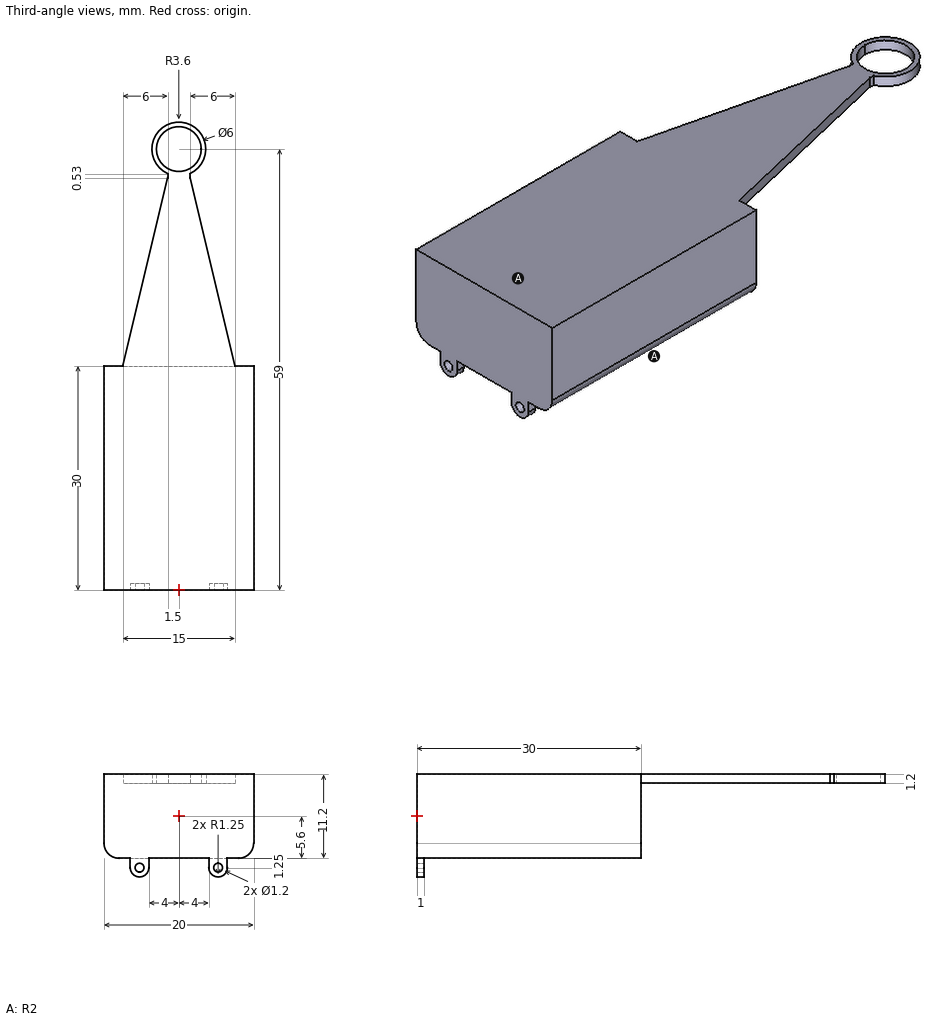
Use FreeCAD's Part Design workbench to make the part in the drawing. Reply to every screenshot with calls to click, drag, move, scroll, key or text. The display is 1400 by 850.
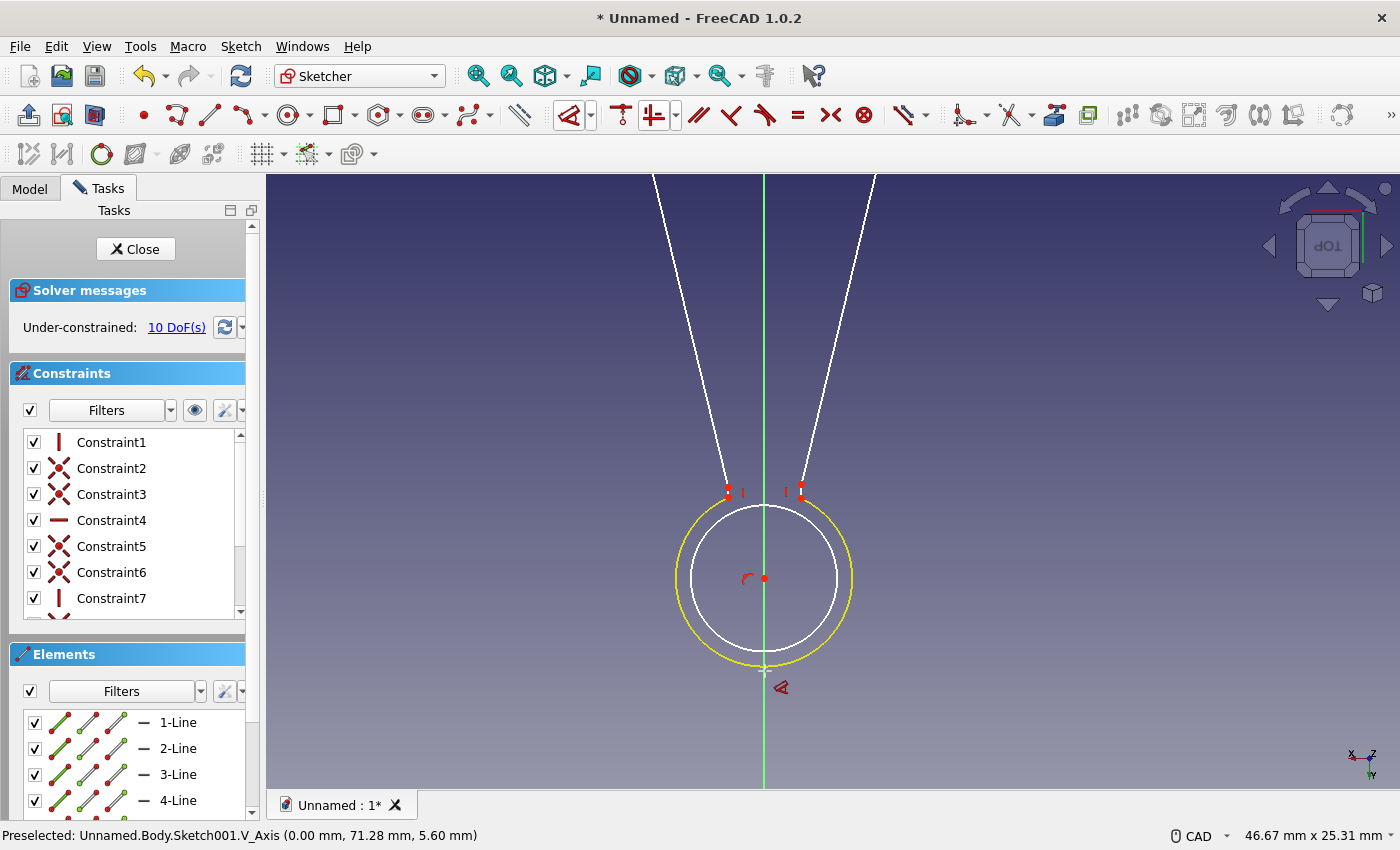
click(763, 667)
click(705, 684)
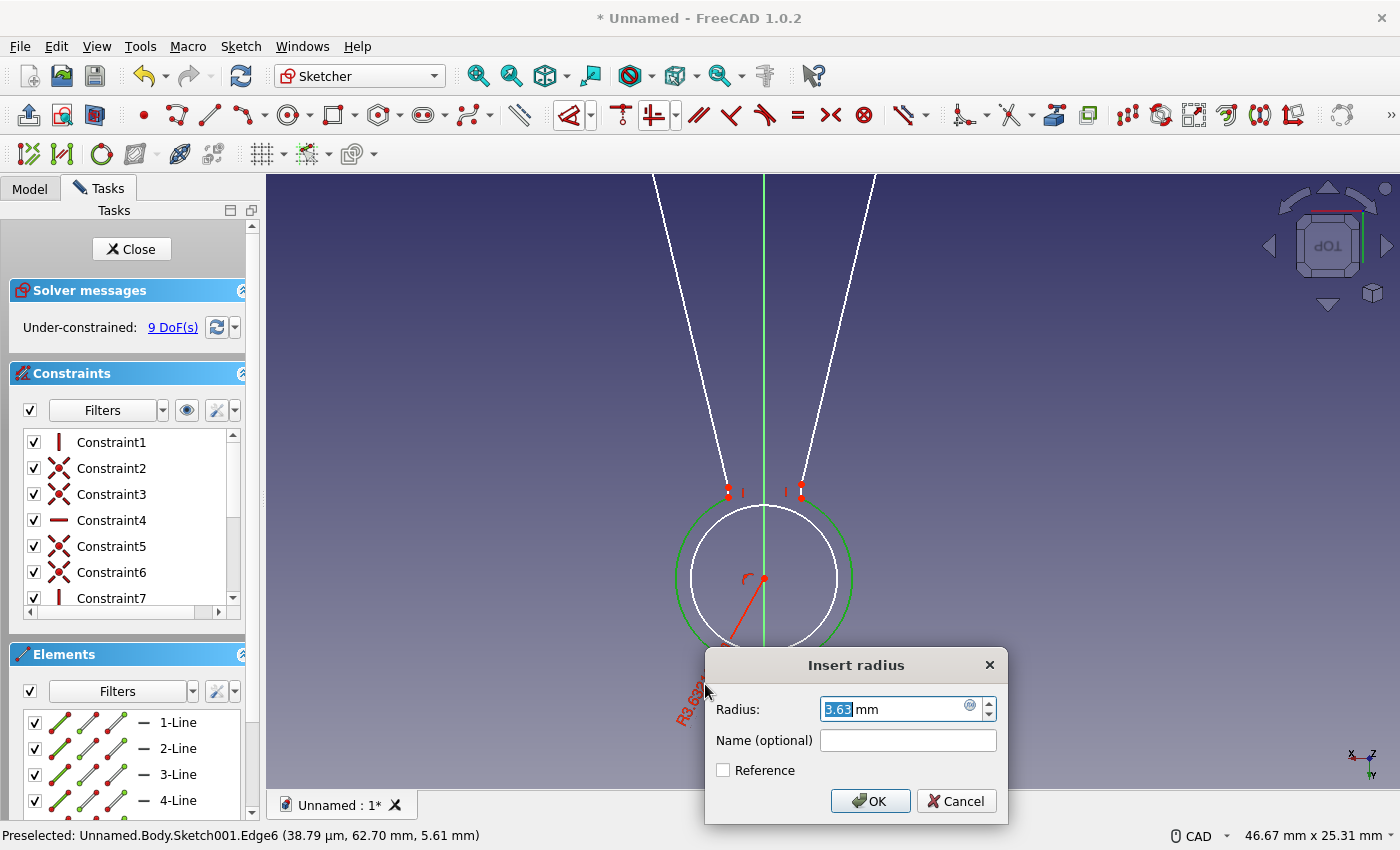
text(3.6)
key(Return)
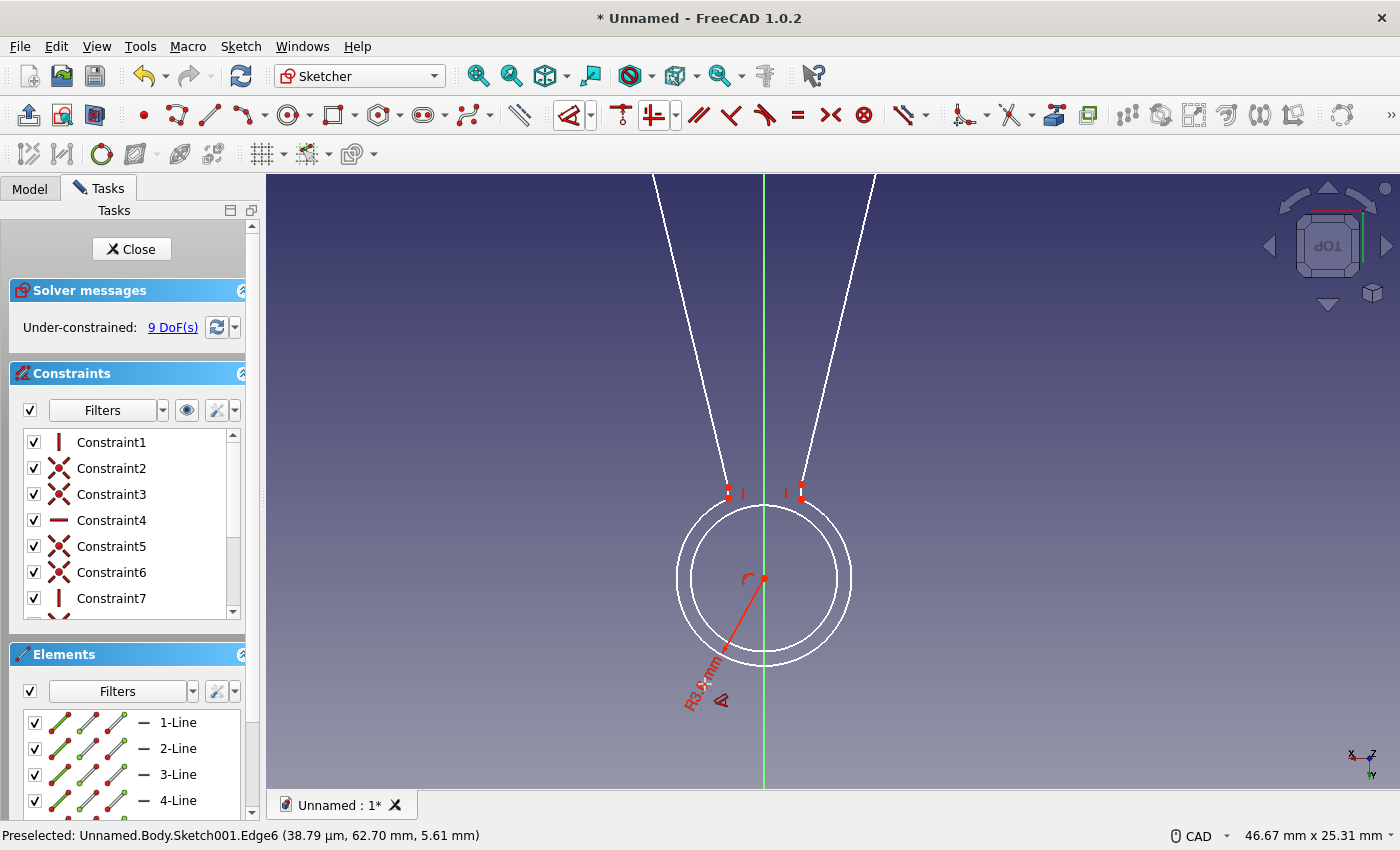
click(816, 527)
click(839, 504)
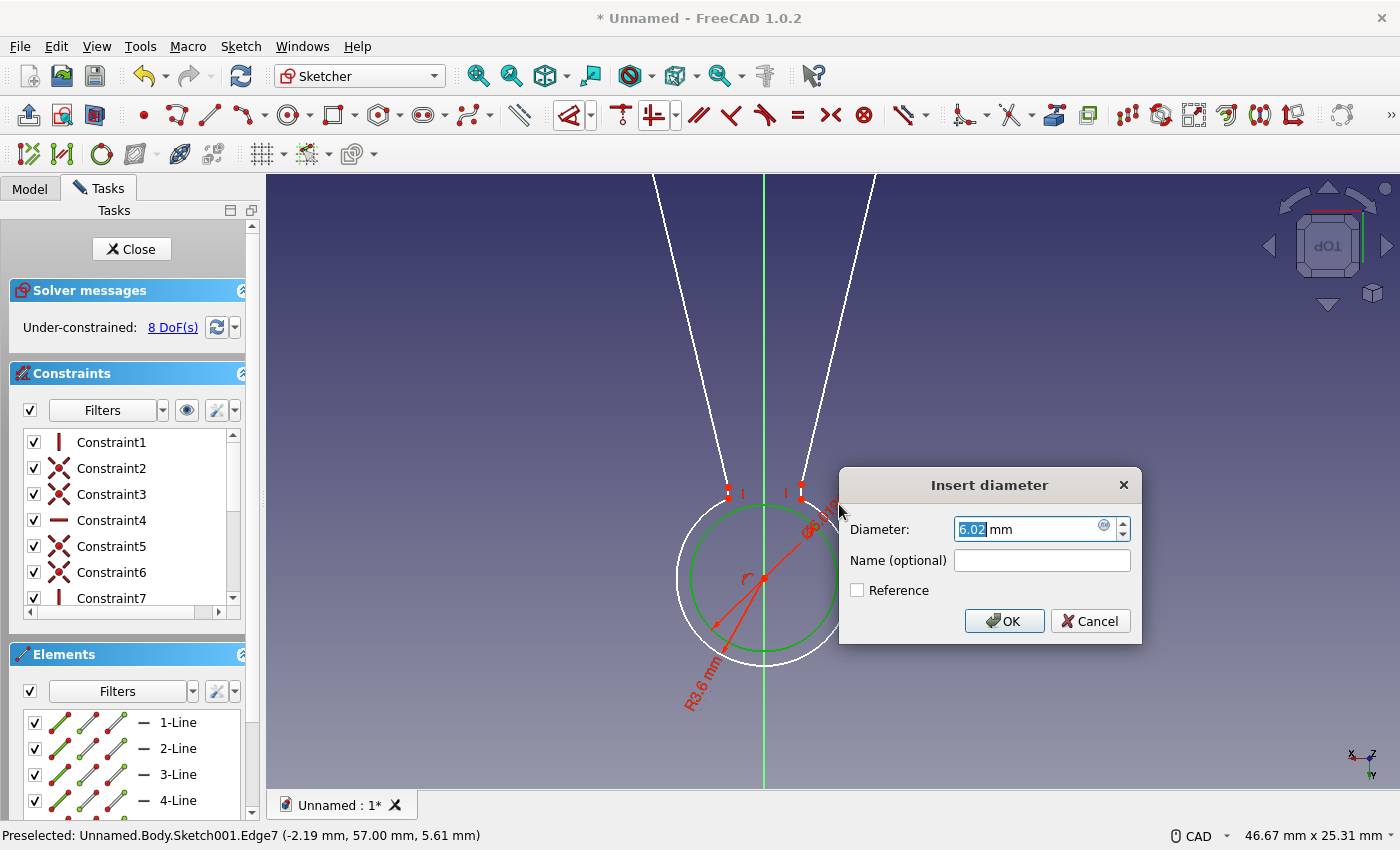
text(6)
key(Return)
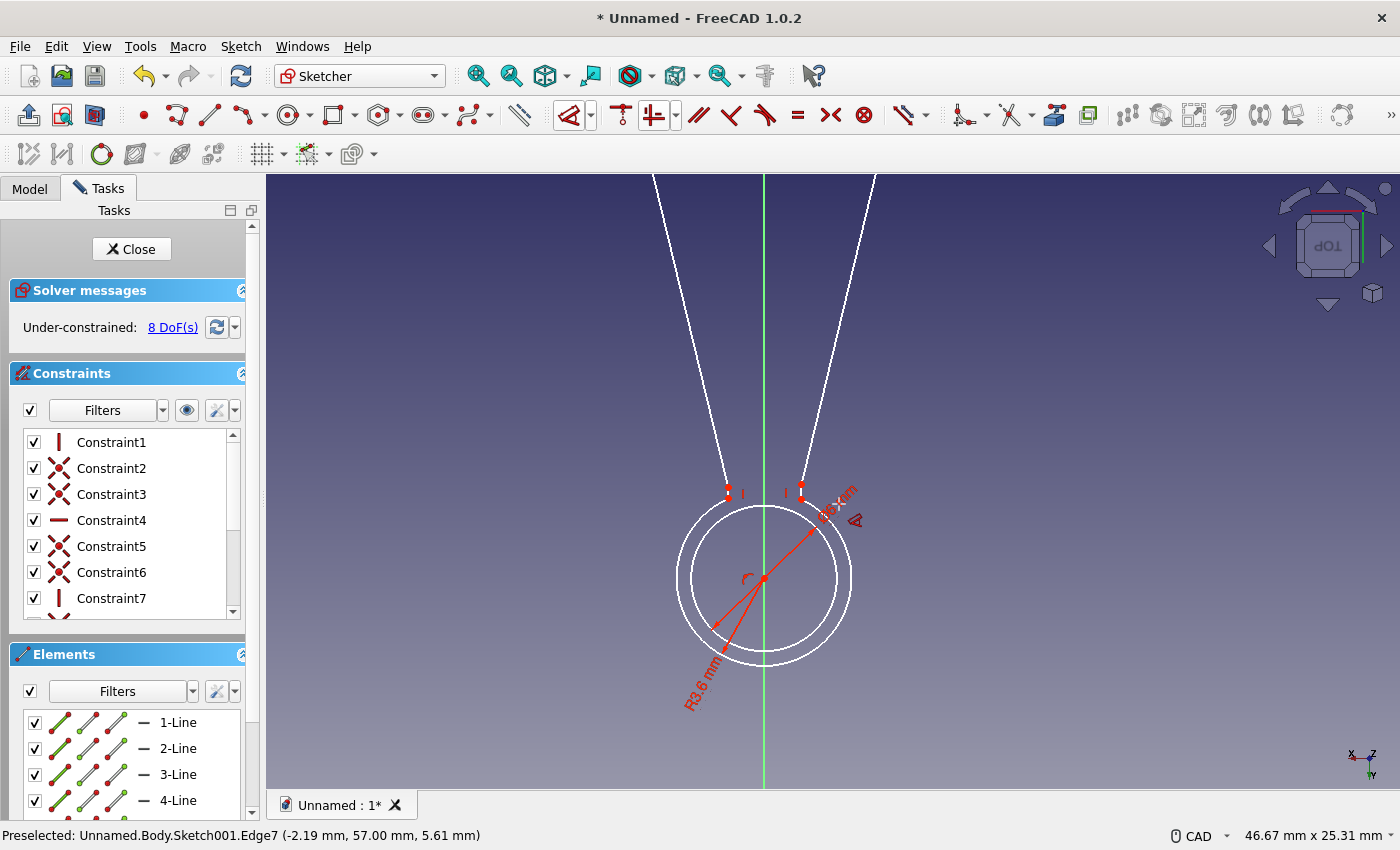
scroll(765, 671, down, 7)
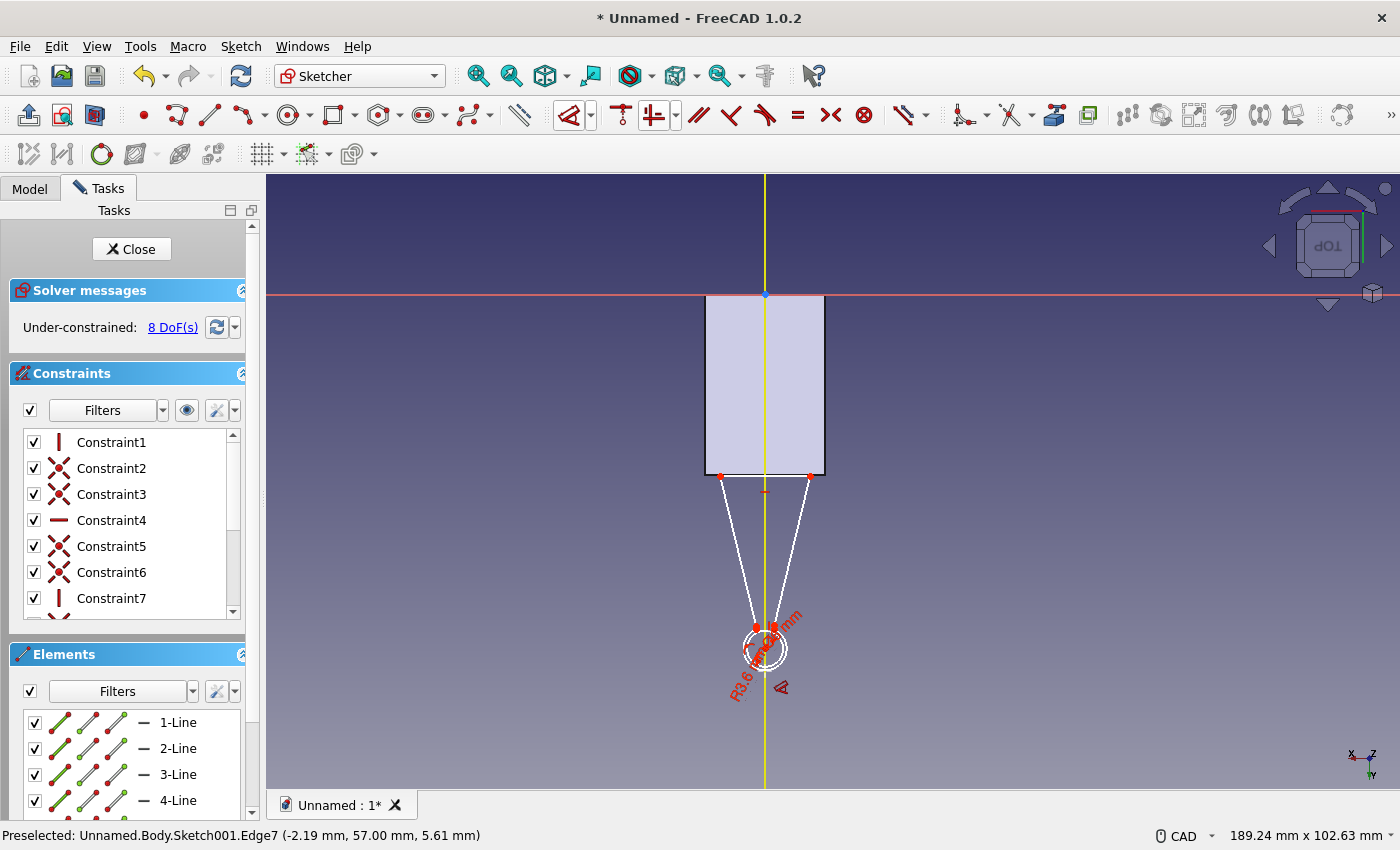
click(783, 476)
click(744, 442)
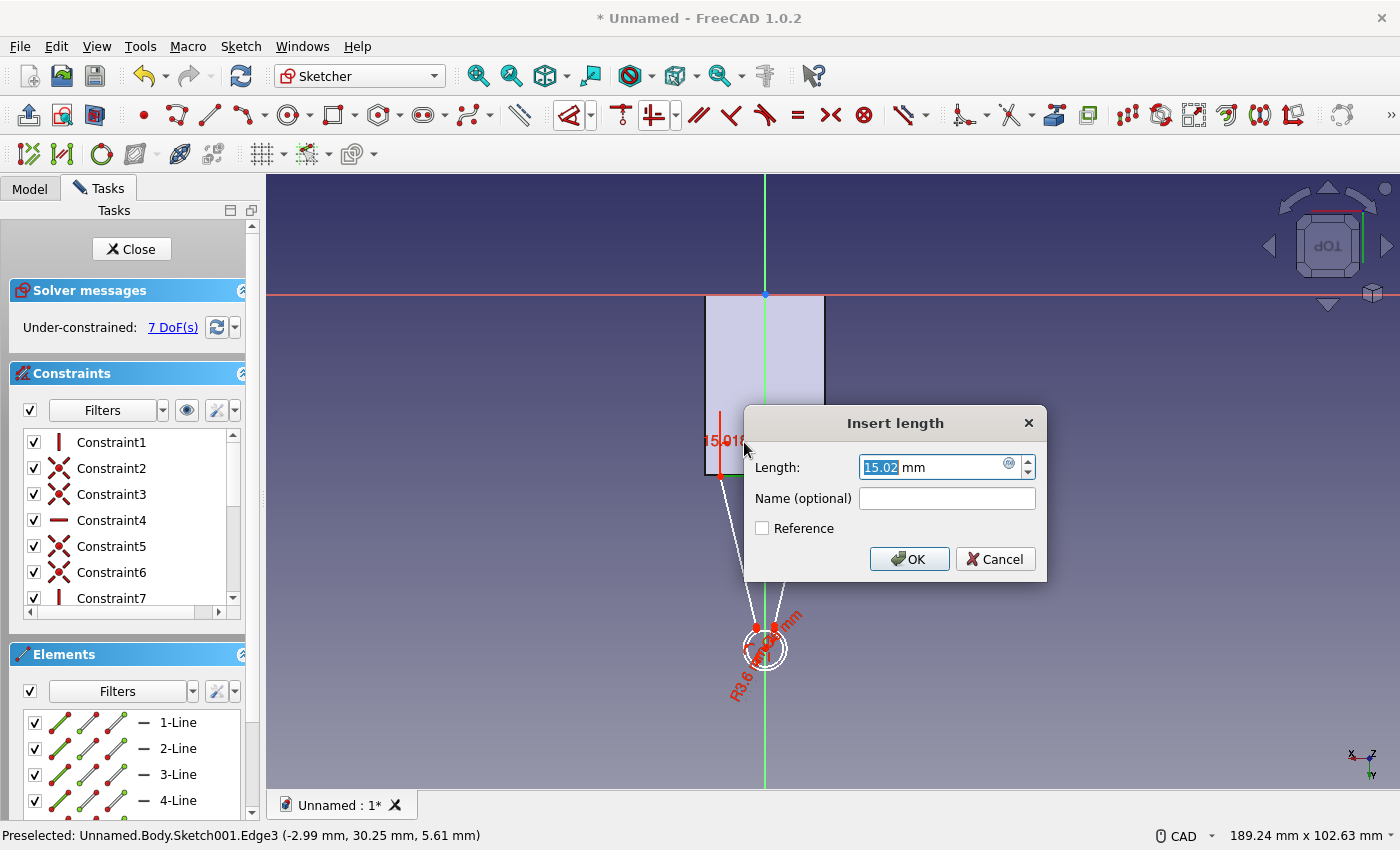
text(15)
key(Return)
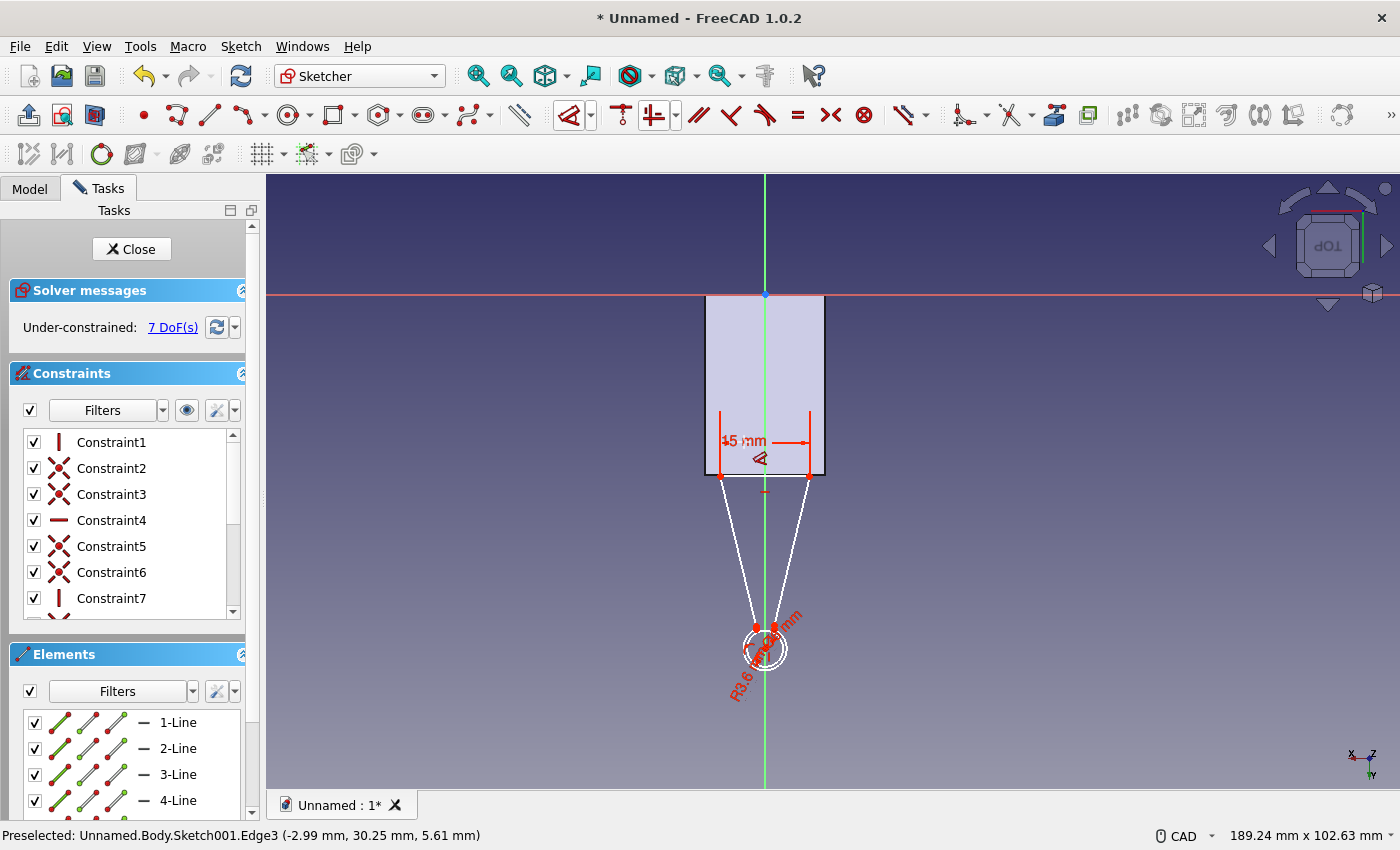
click(785, 581)
click(792, 418)